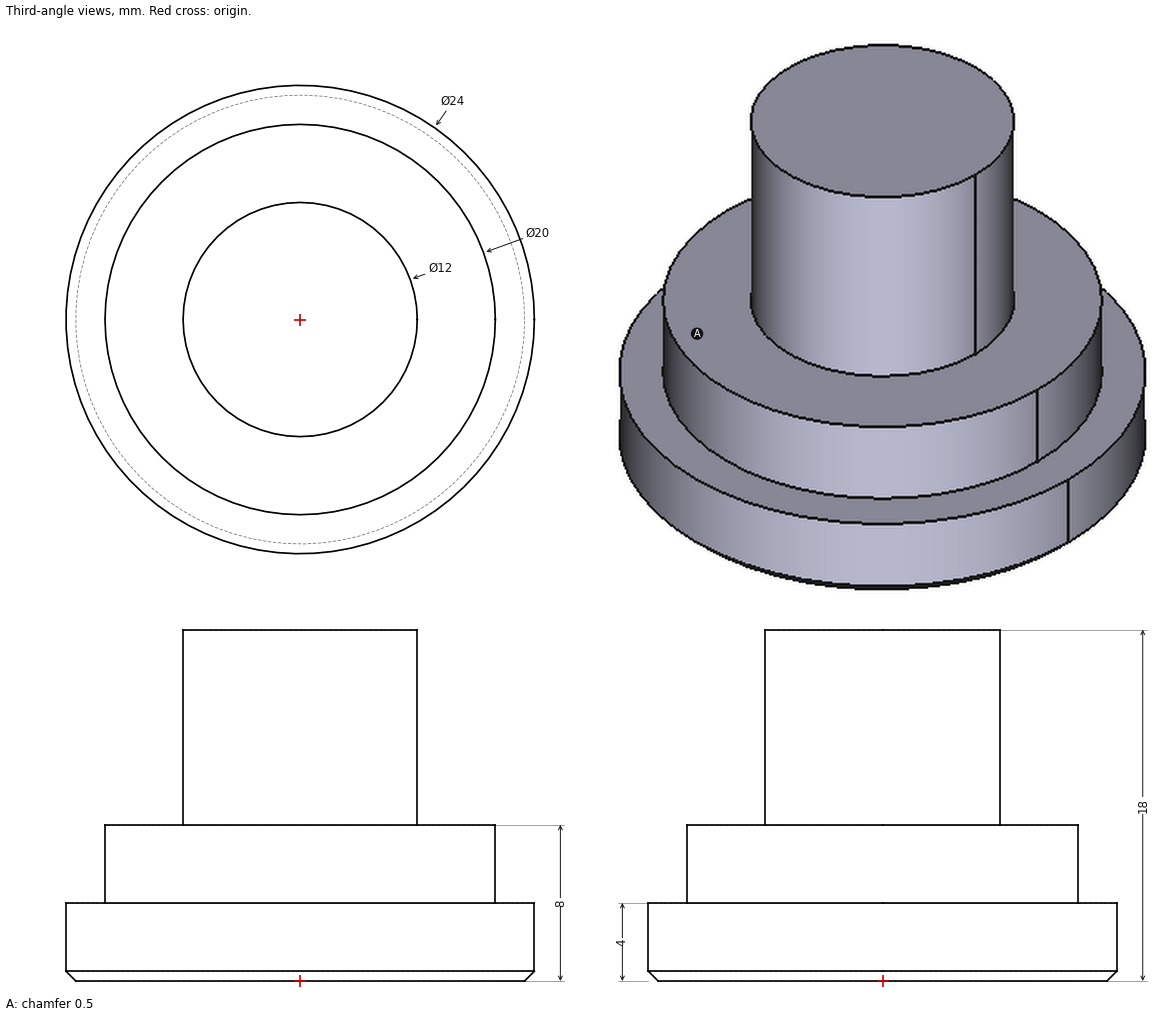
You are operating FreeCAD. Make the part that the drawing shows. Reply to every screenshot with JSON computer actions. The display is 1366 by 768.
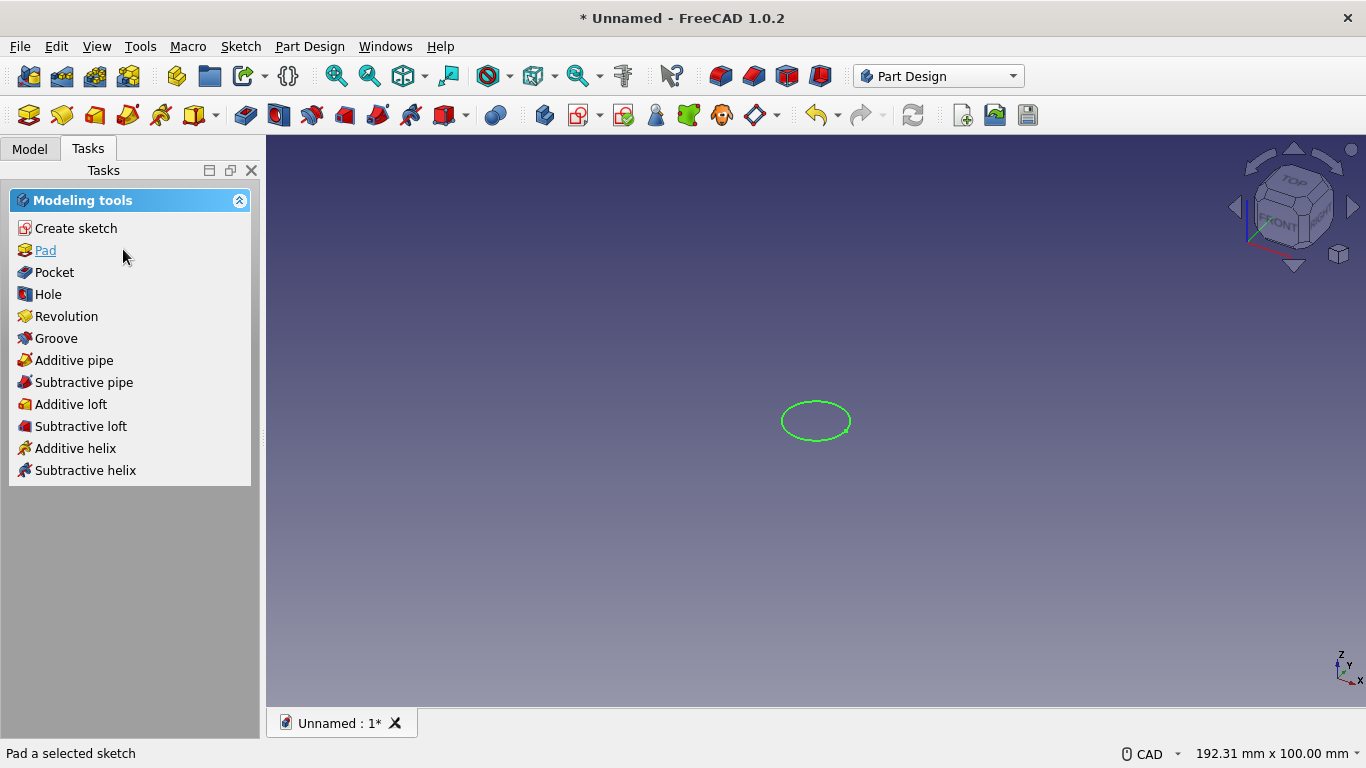
{"action": "left_click", "coordinate": [29, 116]}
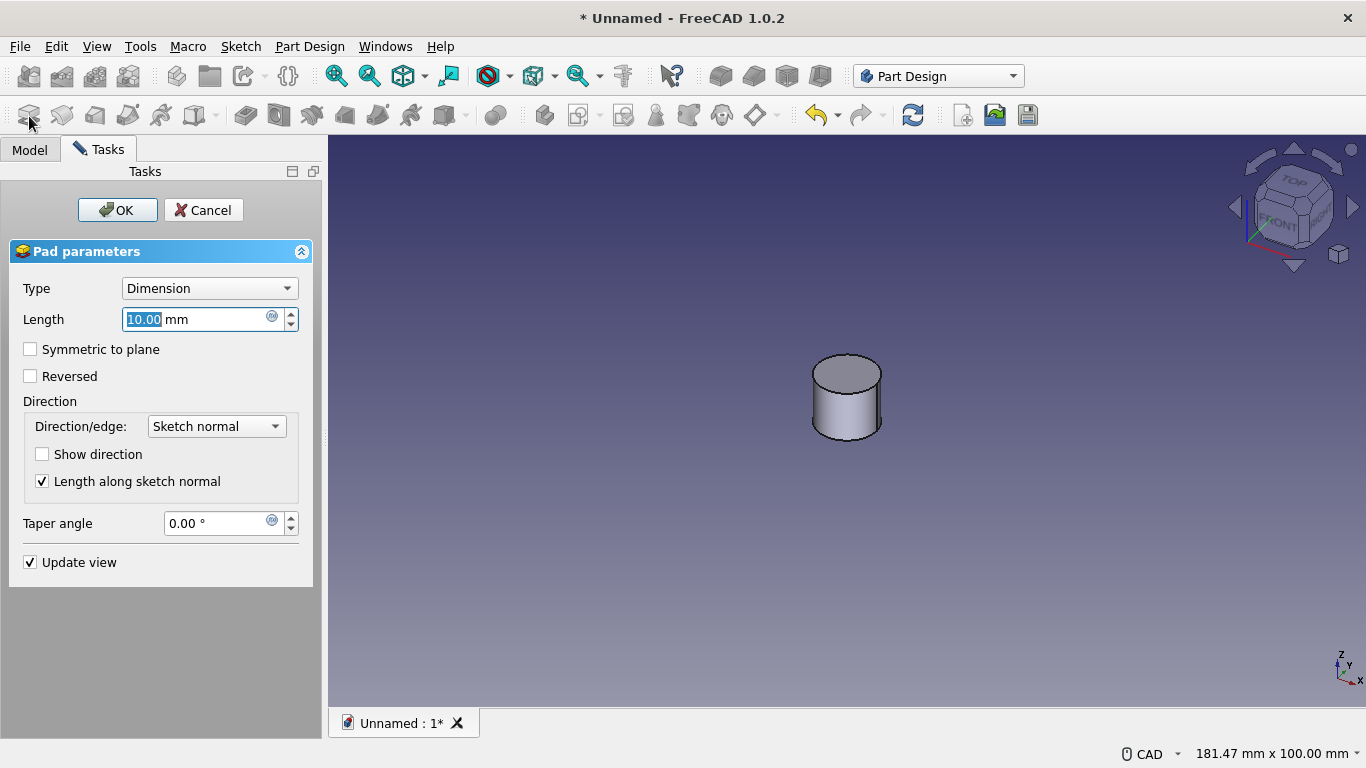
{"action": "type", "text": "18"}
{"action": "key", "text": "Tab"}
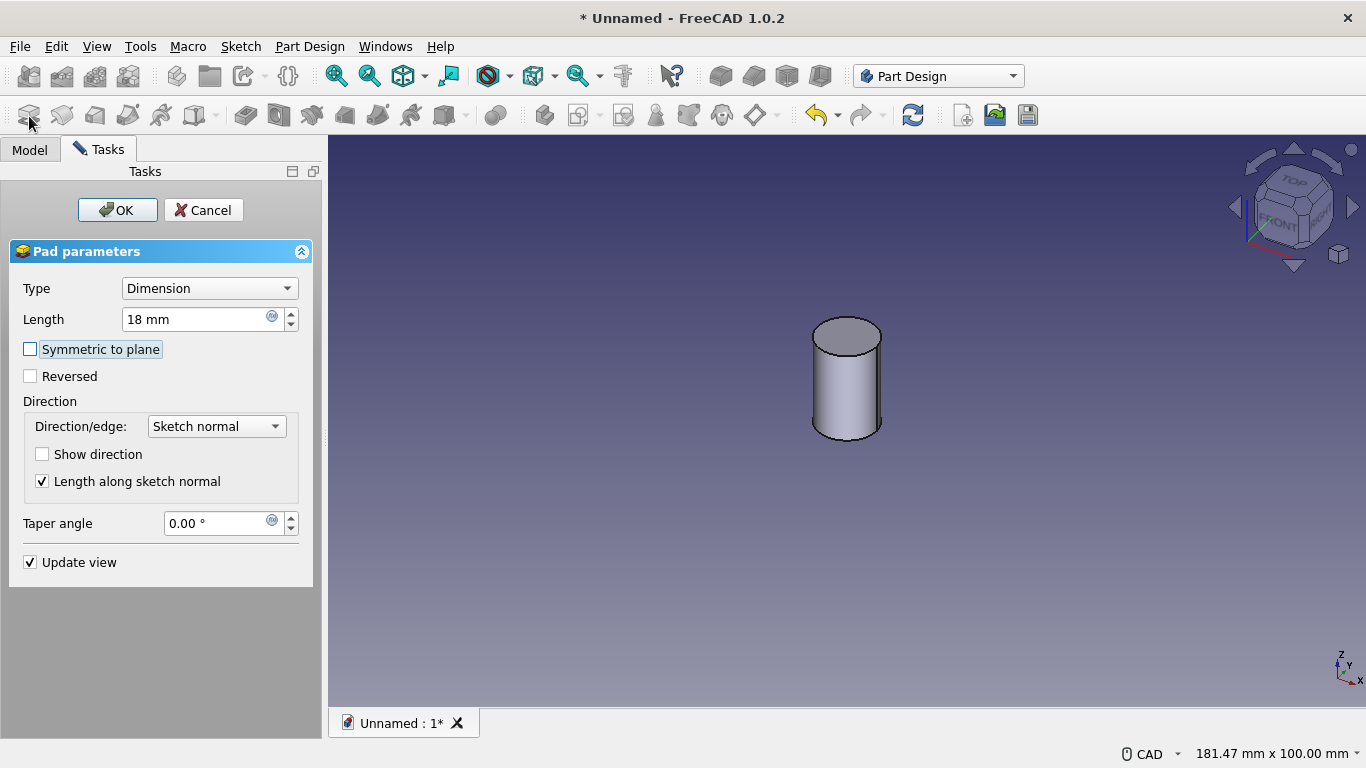
{"action": "left_click", "coordinate": [118, 210]}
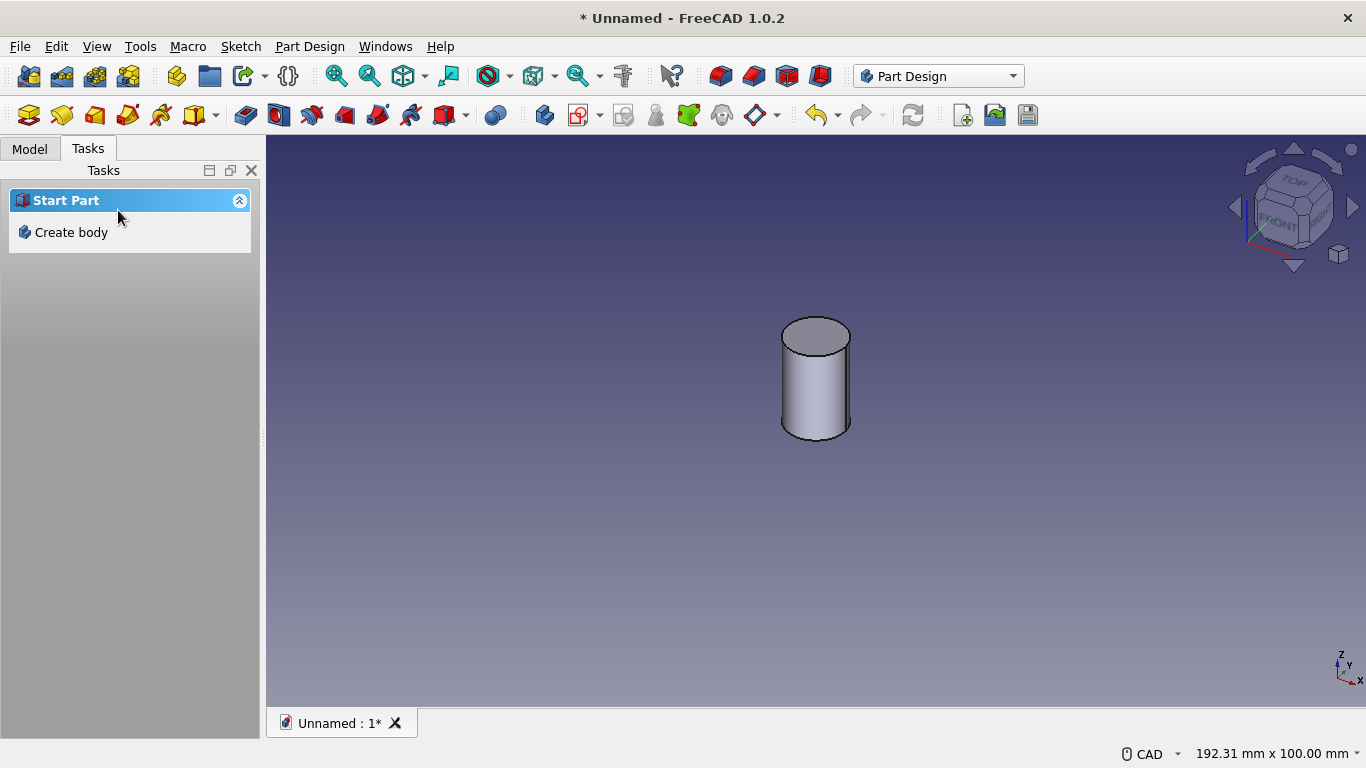
{"action": "left_click", "coordinate": [337, 76]}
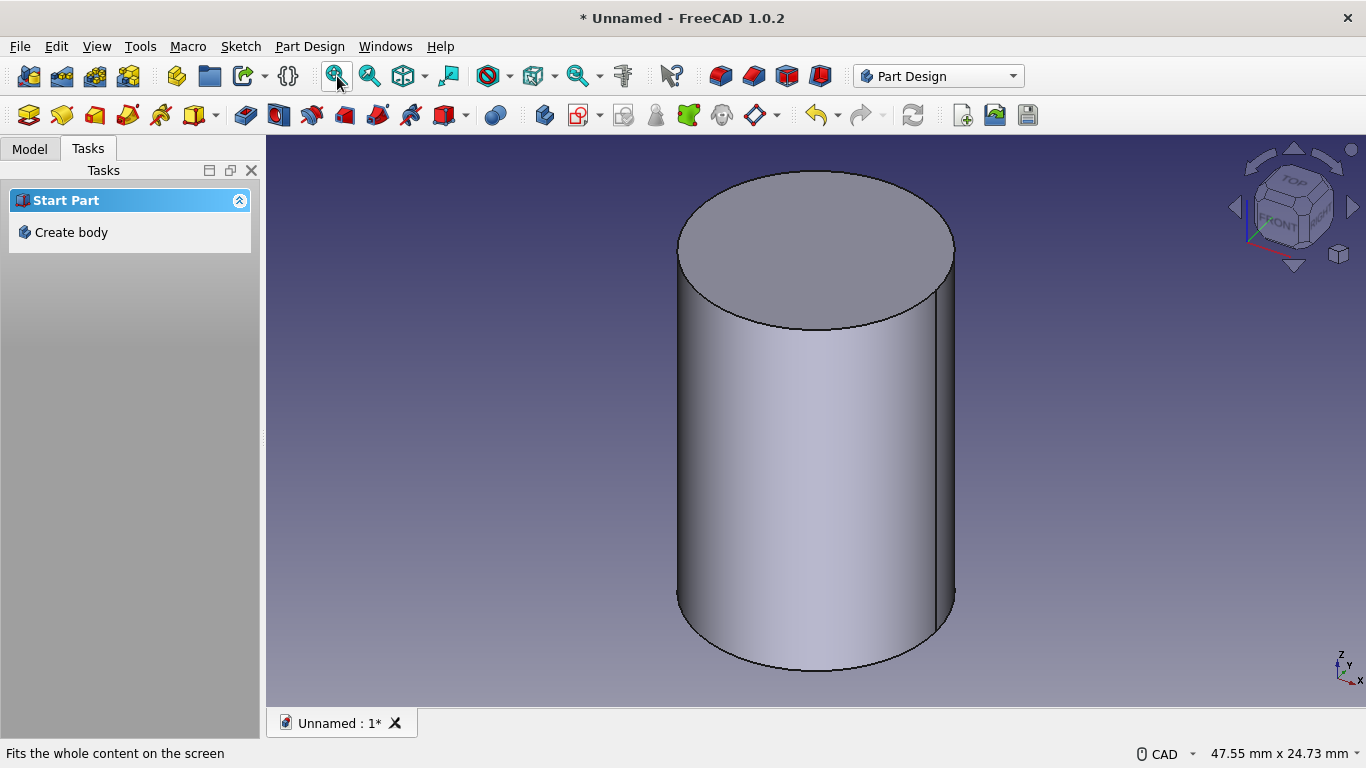
{"action": "key", "text": "5"}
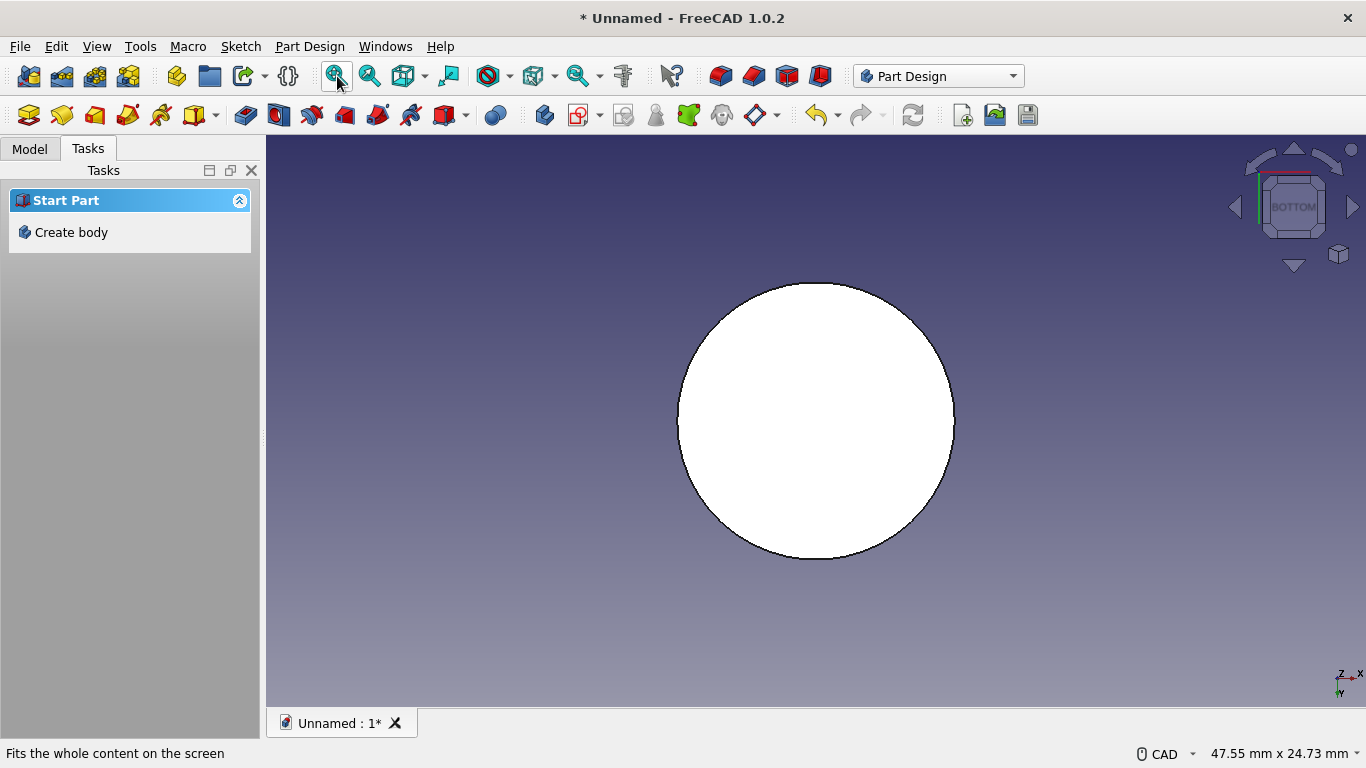
{"action": "left_click", "coordinate": [816, 420]}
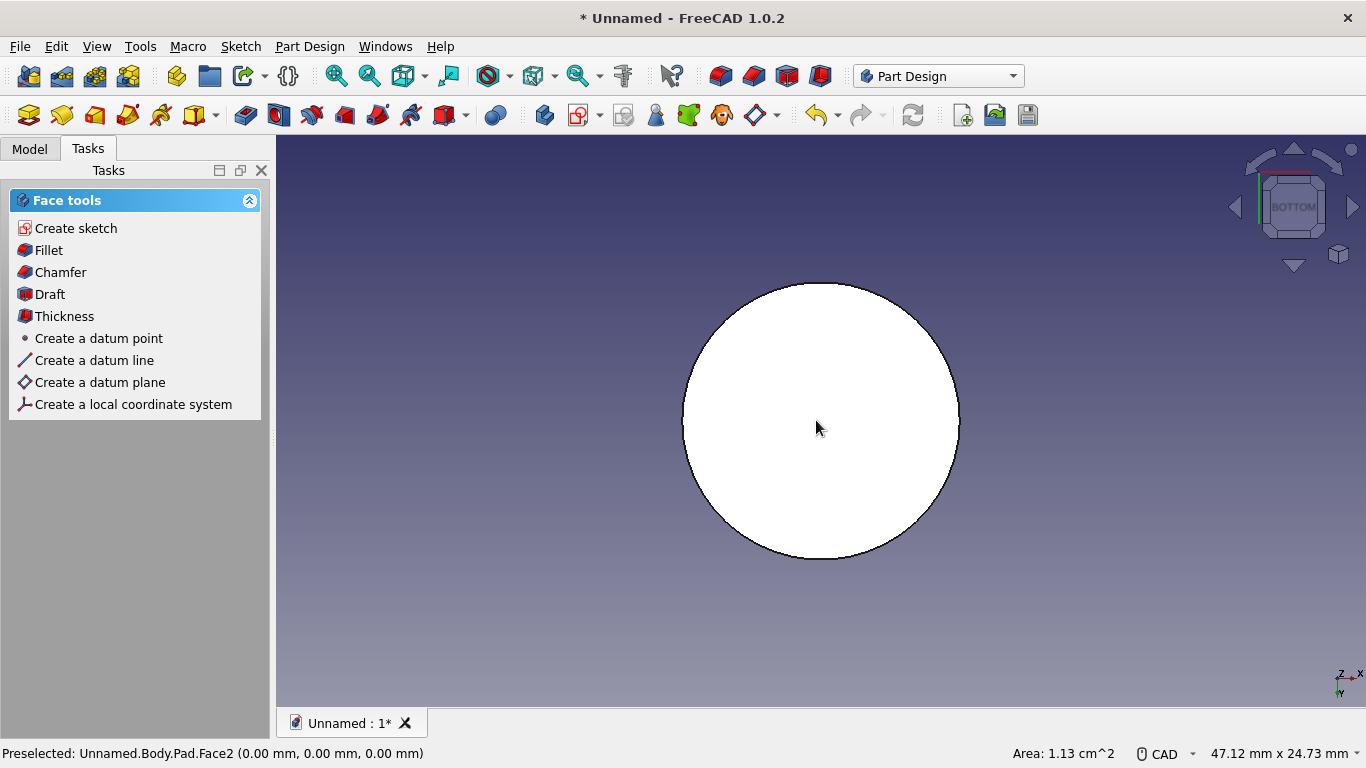
{"action": "left_click", "coordinate": [578, 116]}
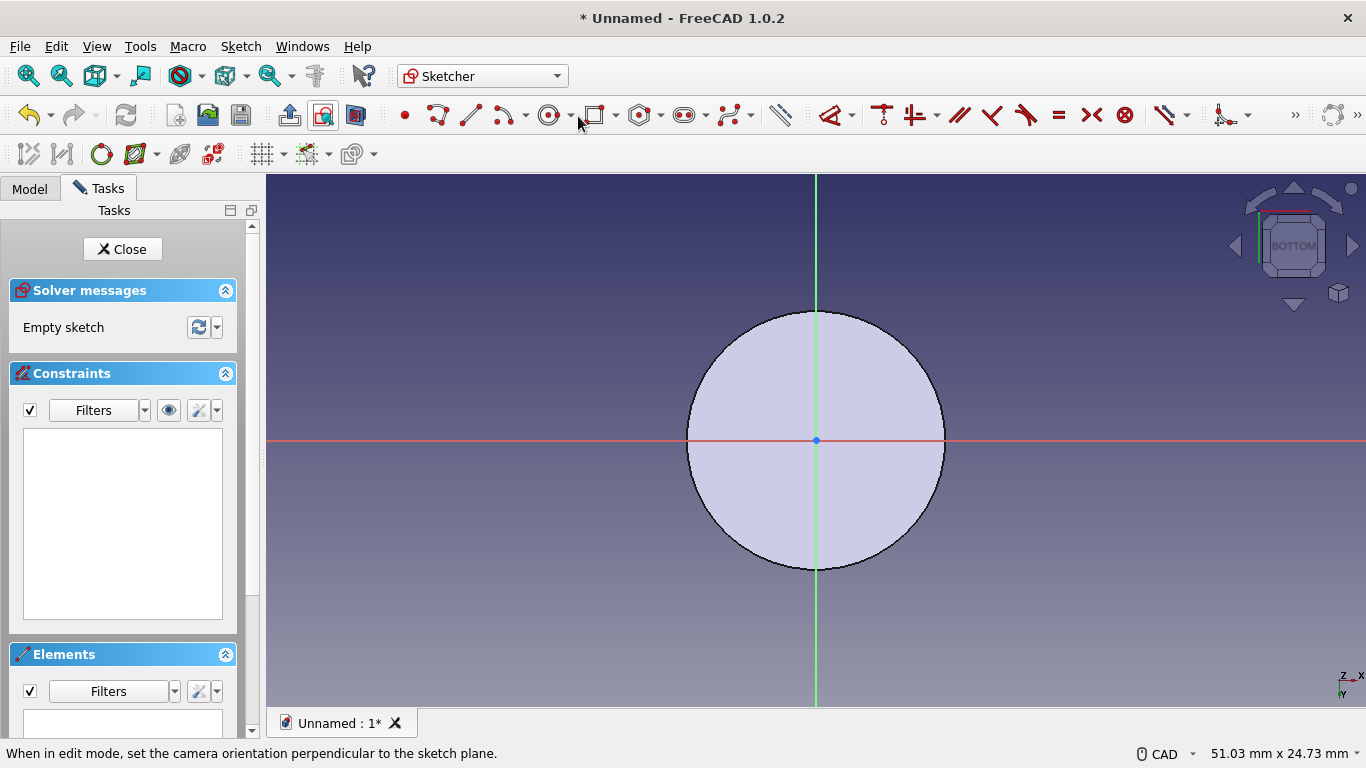
{"action": "scroll", "coordinate": [438, 440], "scroll_direction": "down", "scroll_amount": 1}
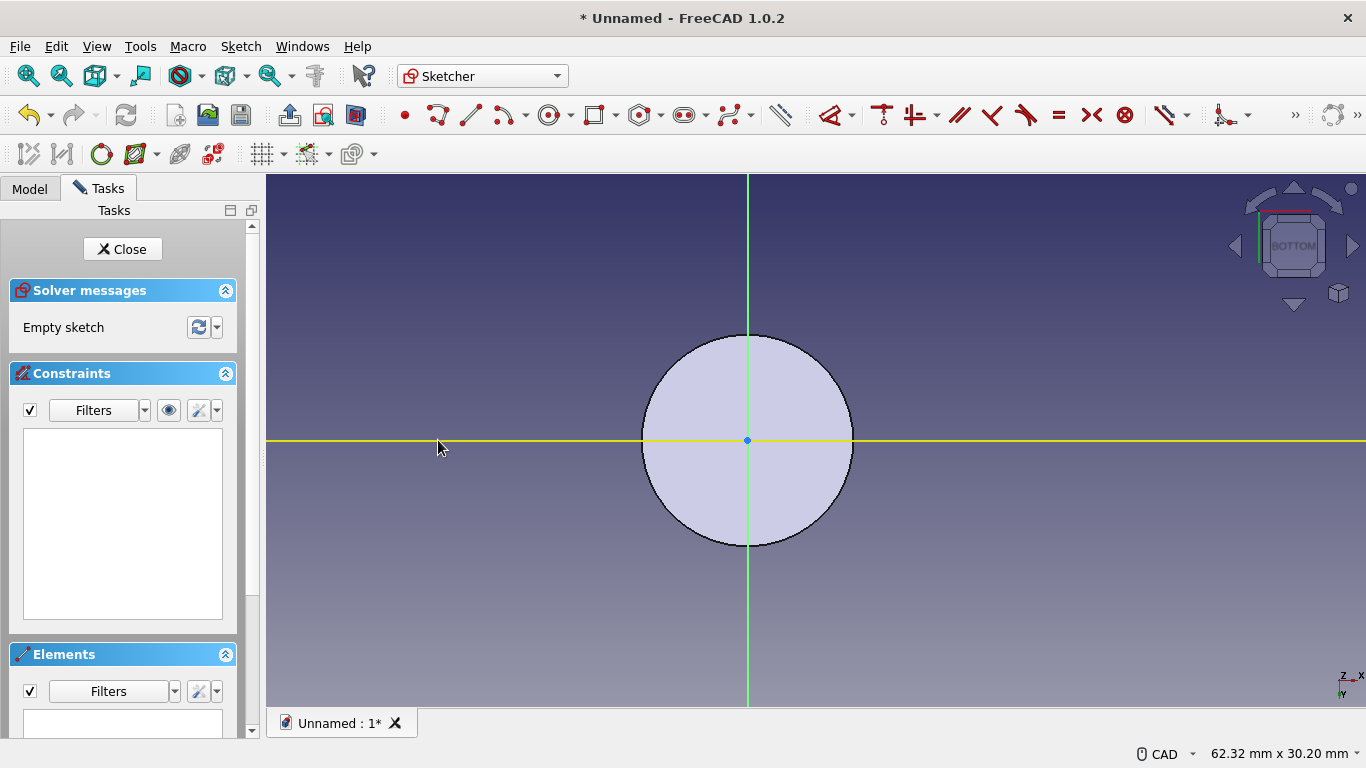
{"action": "left_click", "coordinate": [548, 116]}